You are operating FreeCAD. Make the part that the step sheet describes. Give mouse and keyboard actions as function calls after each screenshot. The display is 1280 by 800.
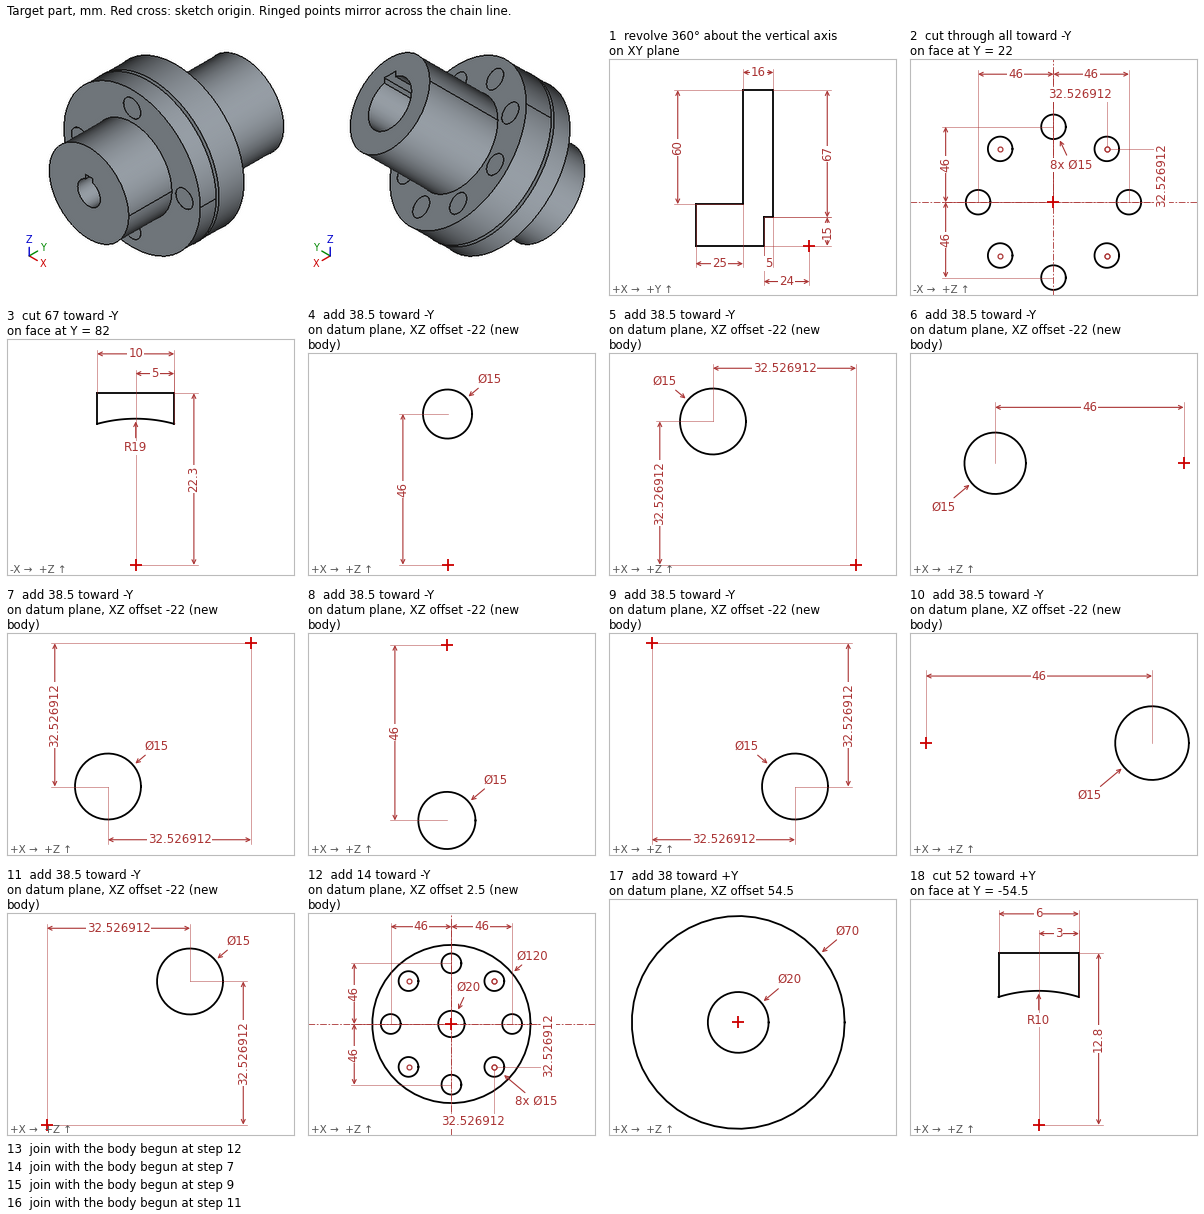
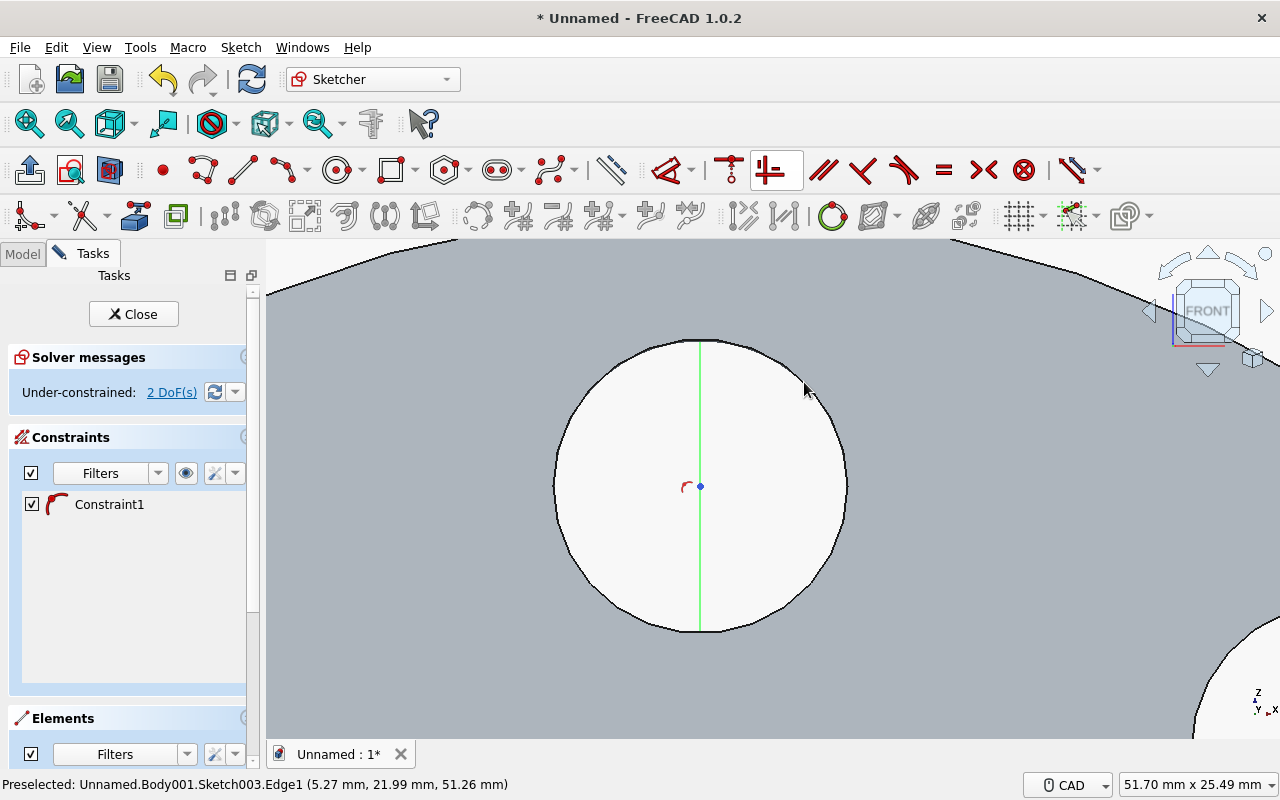
click(666, 170)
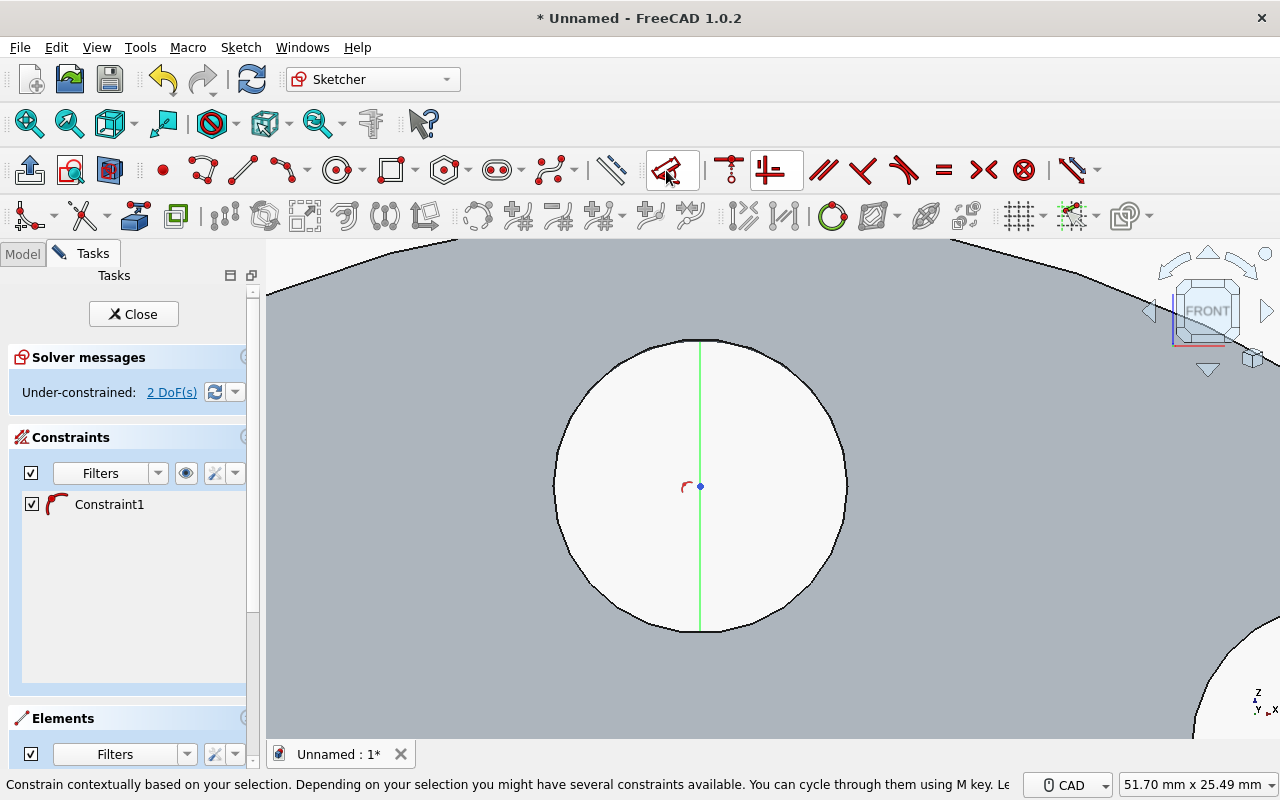
click(804, 383)
click(827, 360)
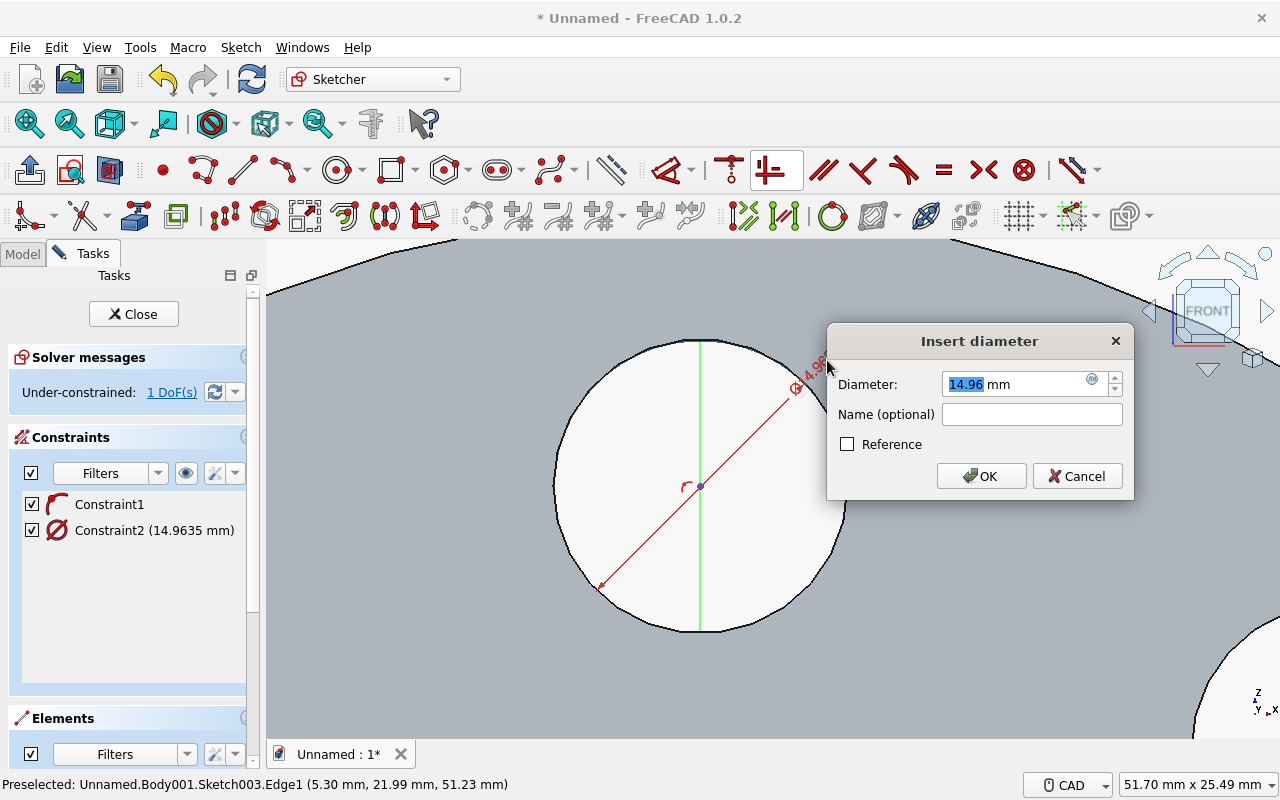
text(15)
key(Return)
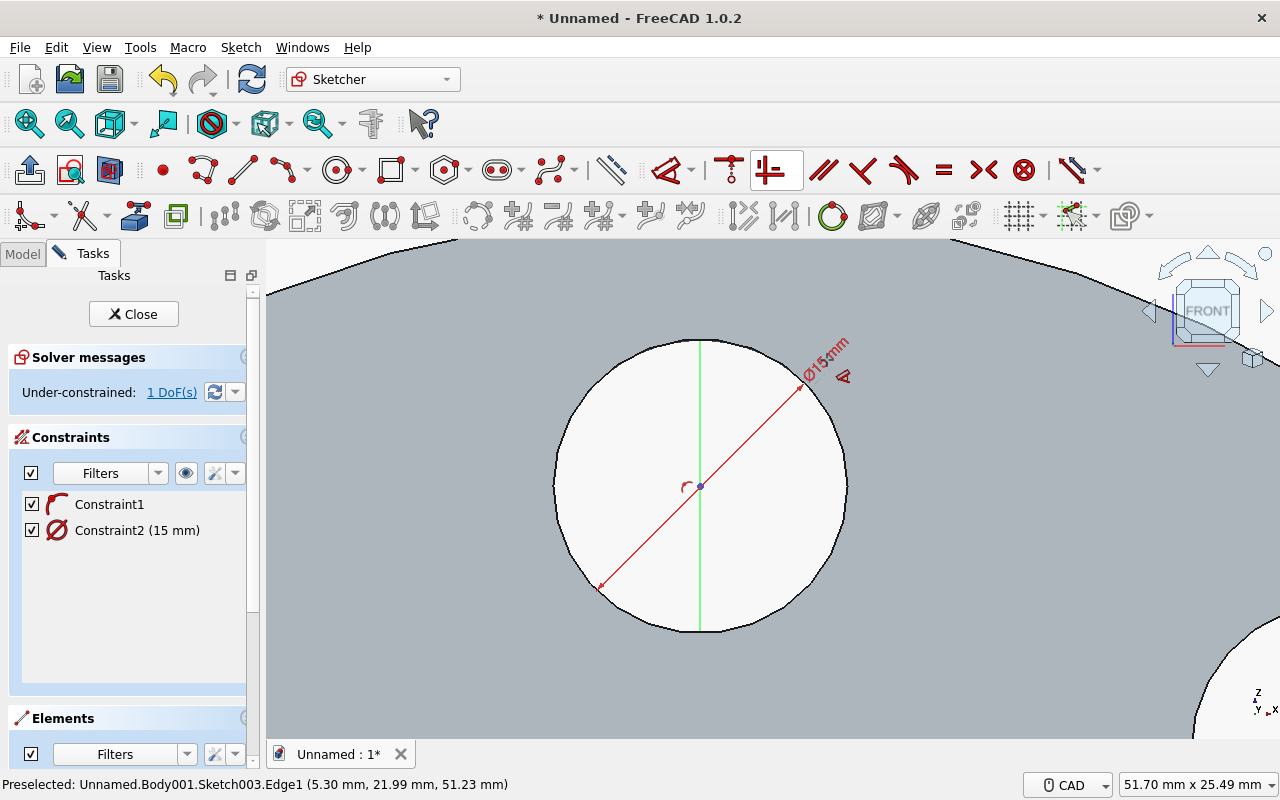
click(700, 487)
click(734, 599)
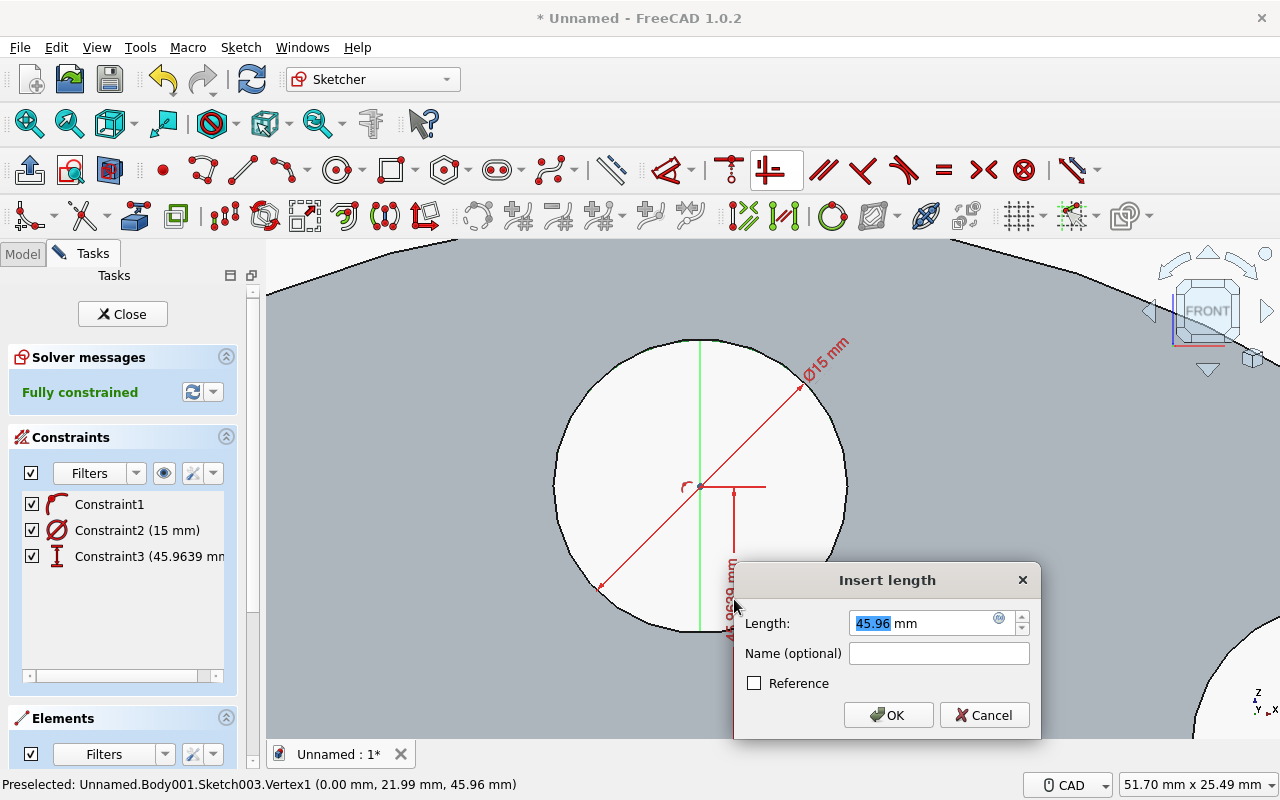
text(46)
key(Return)
key(Escape)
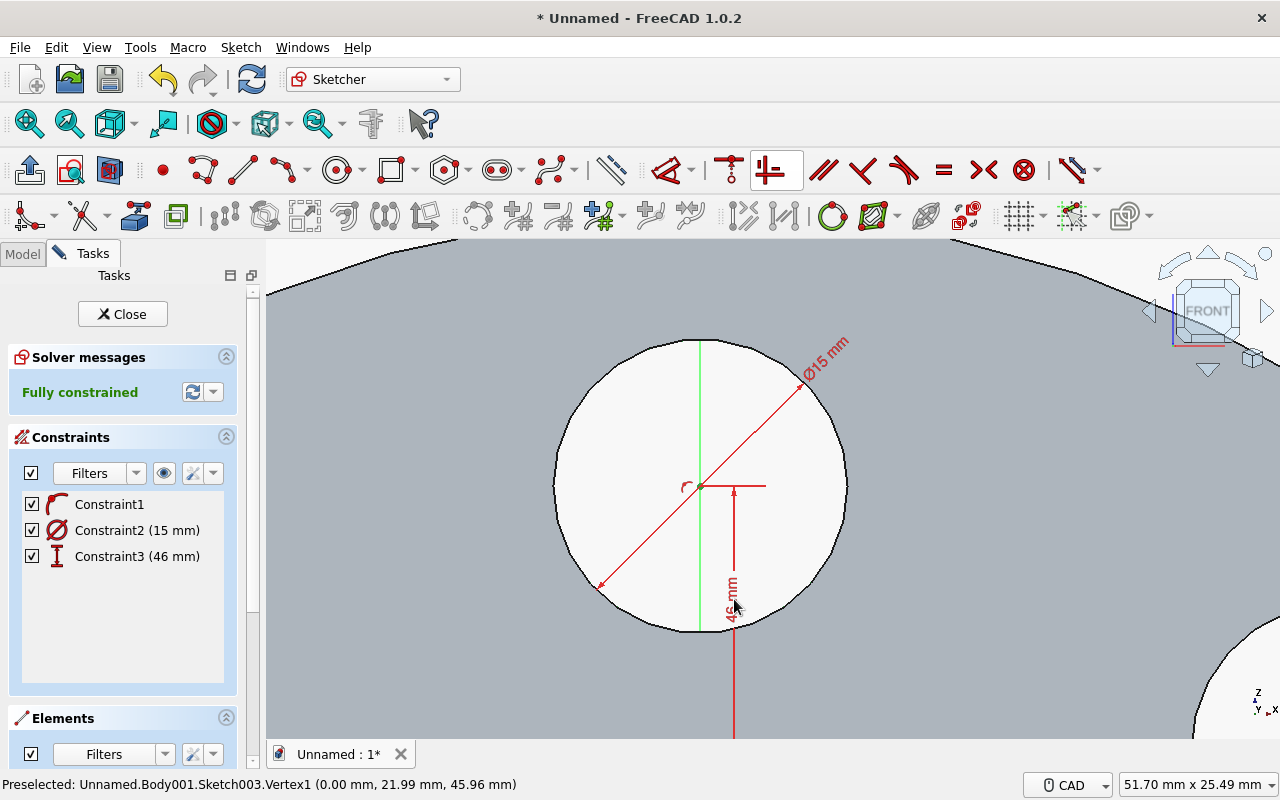
click(123, 314)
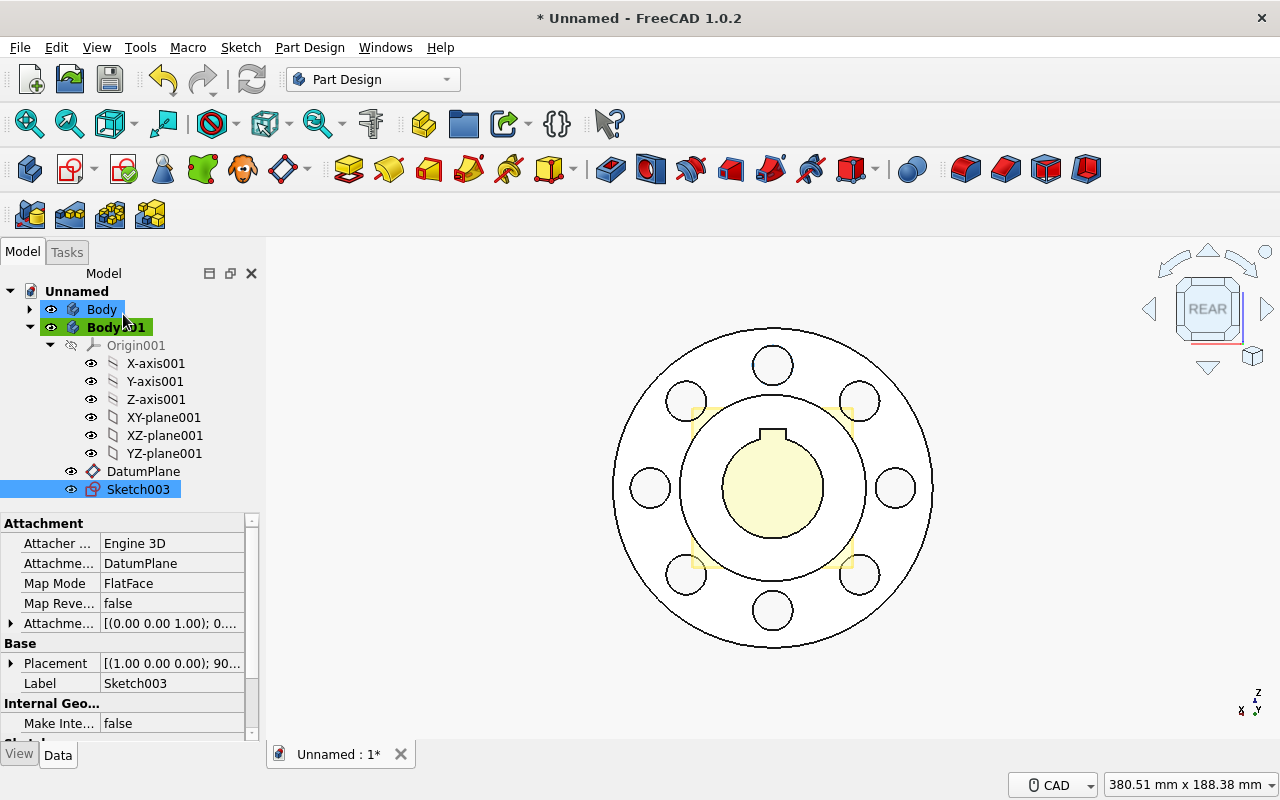
click(350, 170)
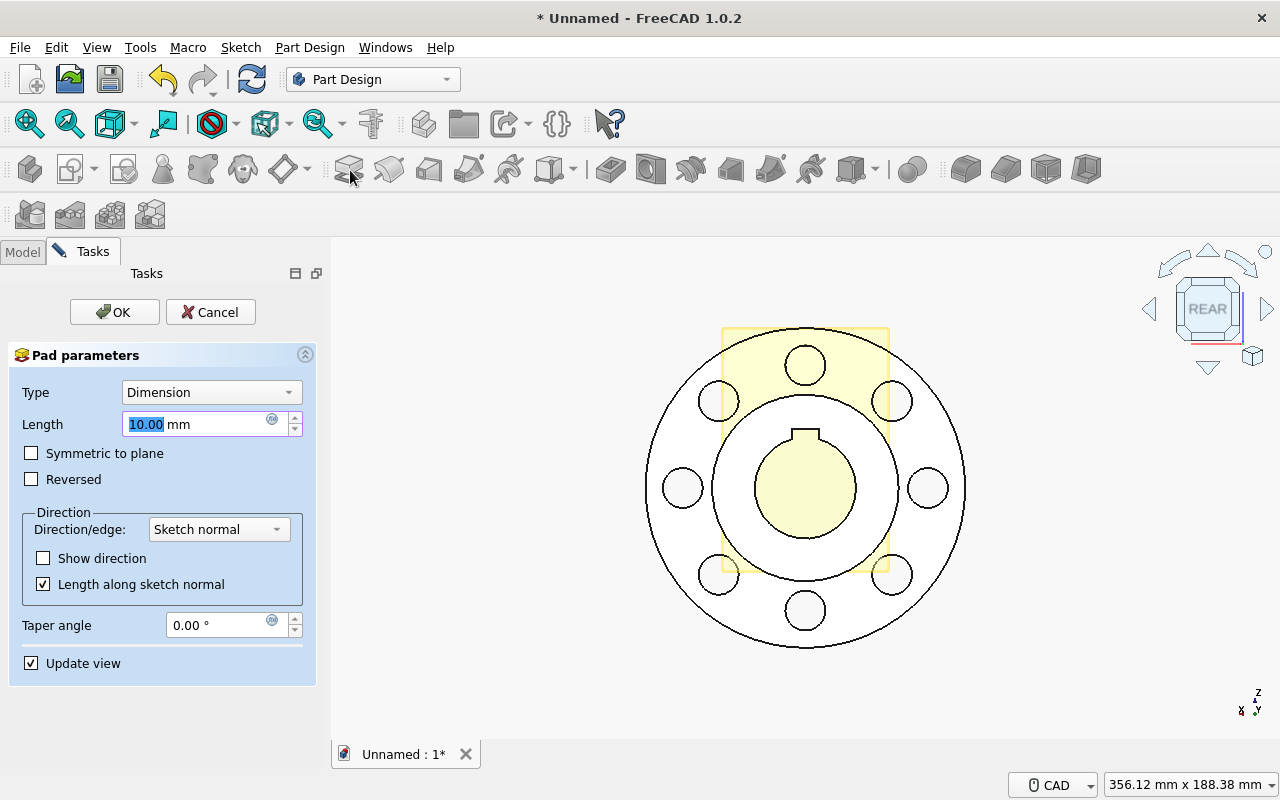
text(38.5)
key(Tab)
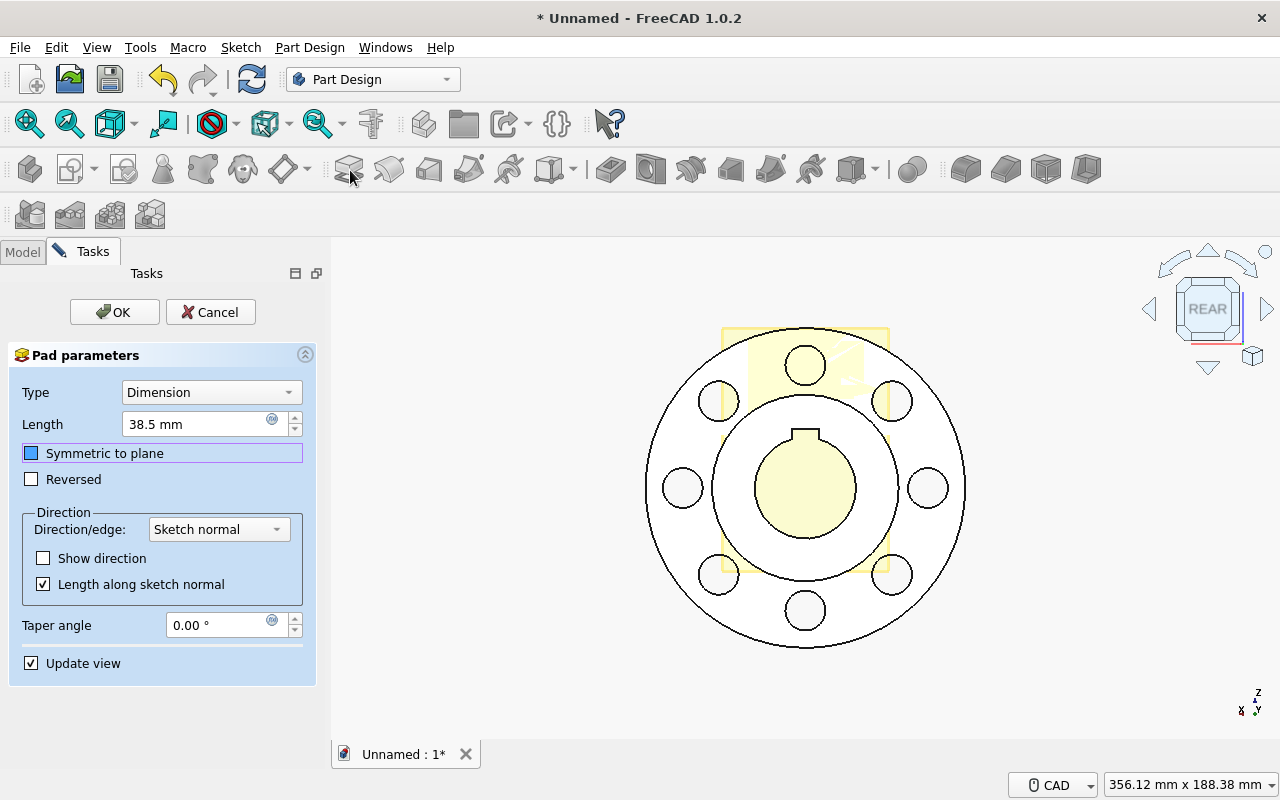
click(115, 312)